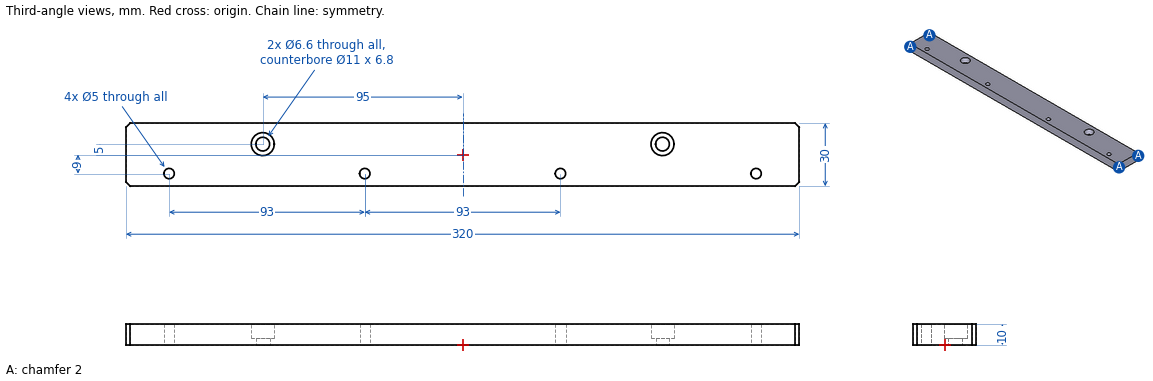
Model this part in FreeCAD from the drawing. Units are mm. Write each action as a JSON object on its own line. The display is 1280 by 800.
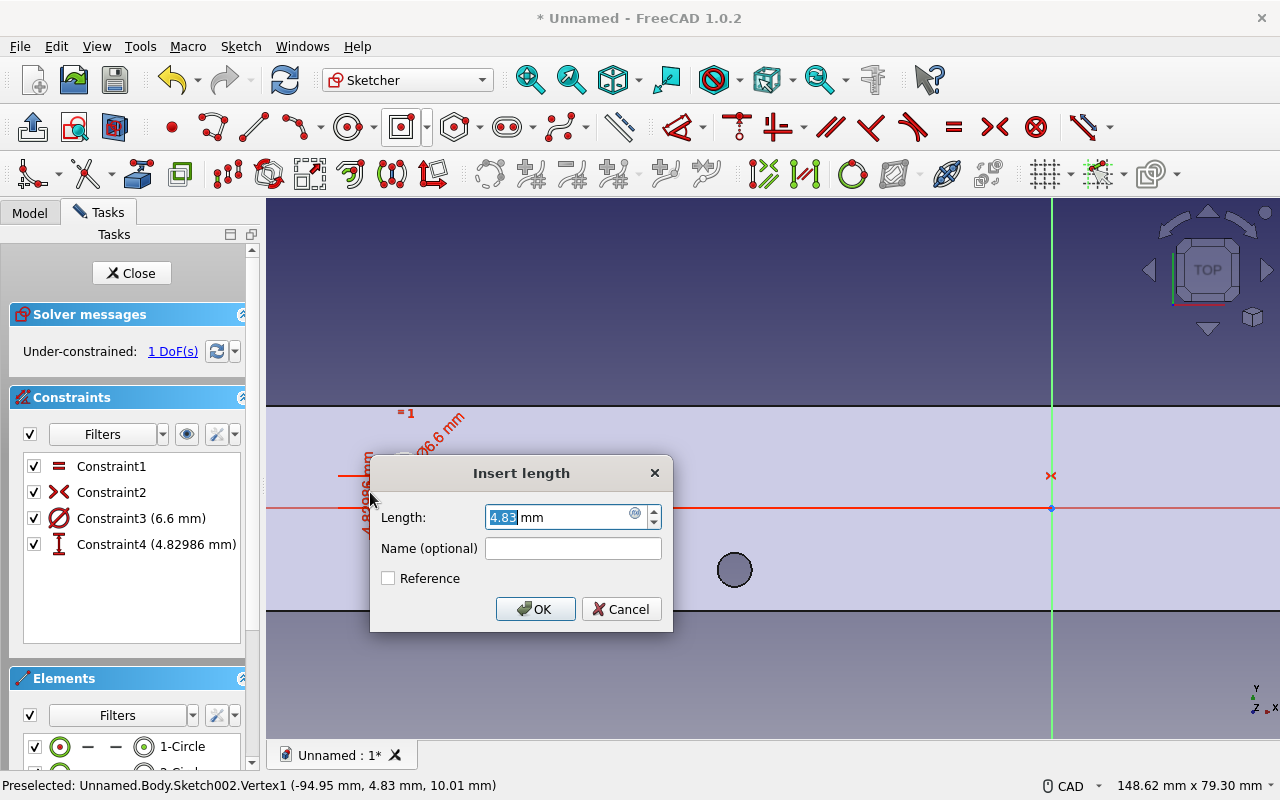
{"action": "type", "text": "5"}
{"action": "key", "text": "Return"}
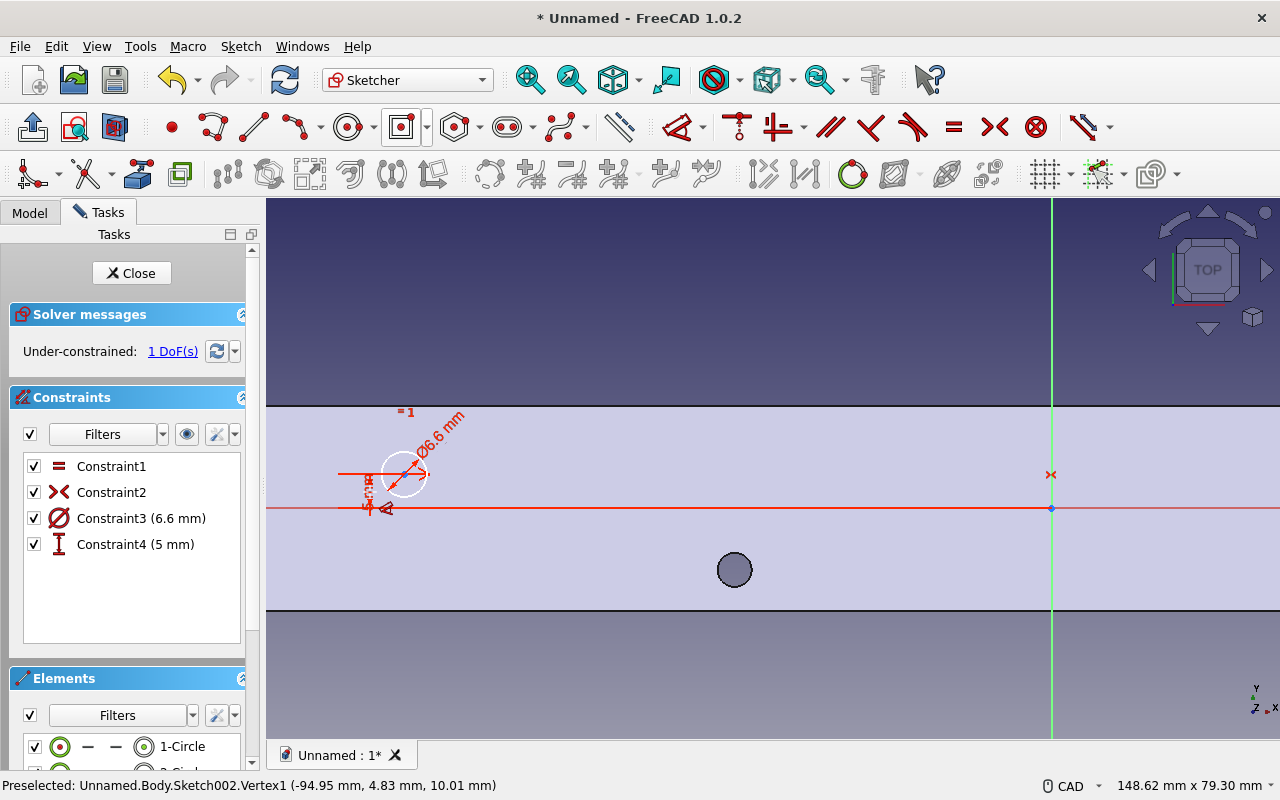
{"action": "left_click", "coordinate": [404, 474]}
{"action": "left_click", "coordinate": [728, 542]}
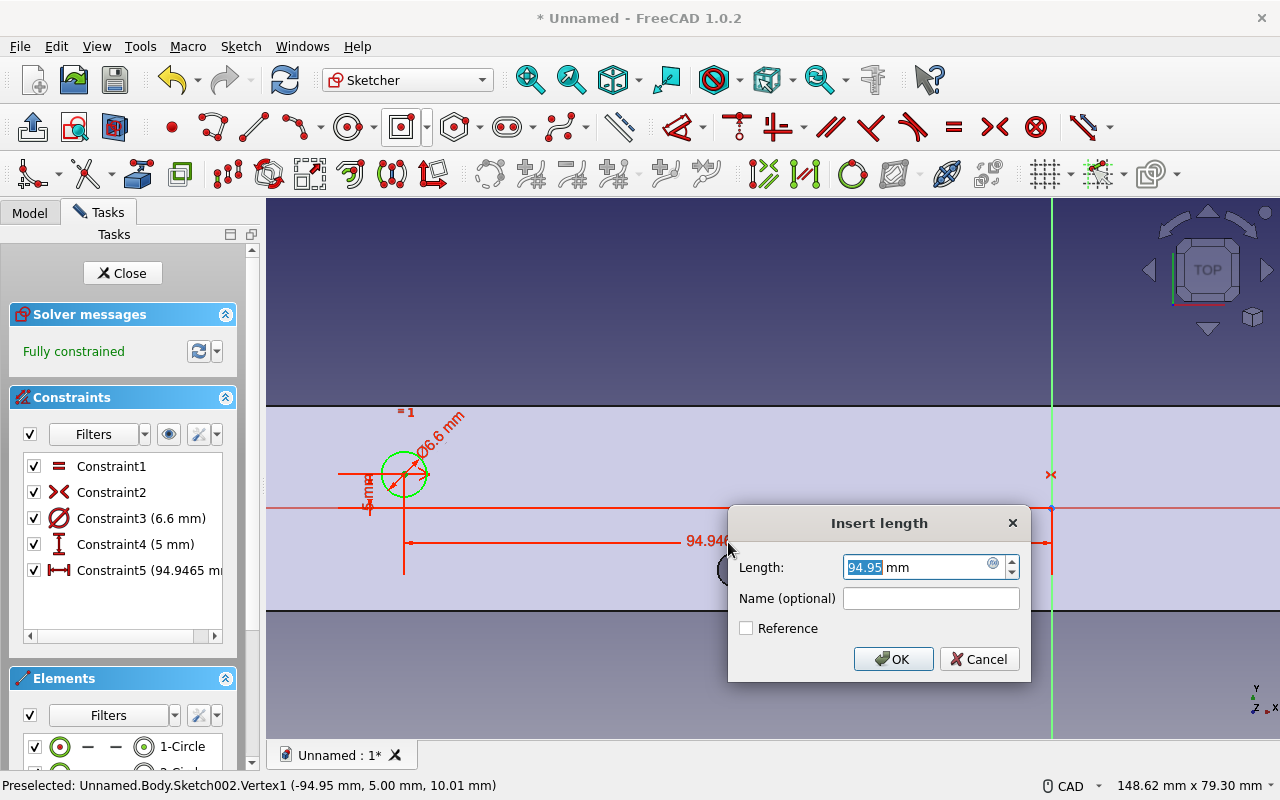
{"action": "type", "text": "95"}
{"action": "key", "text": "Return"}
{"action": "key", "text": "Escape"}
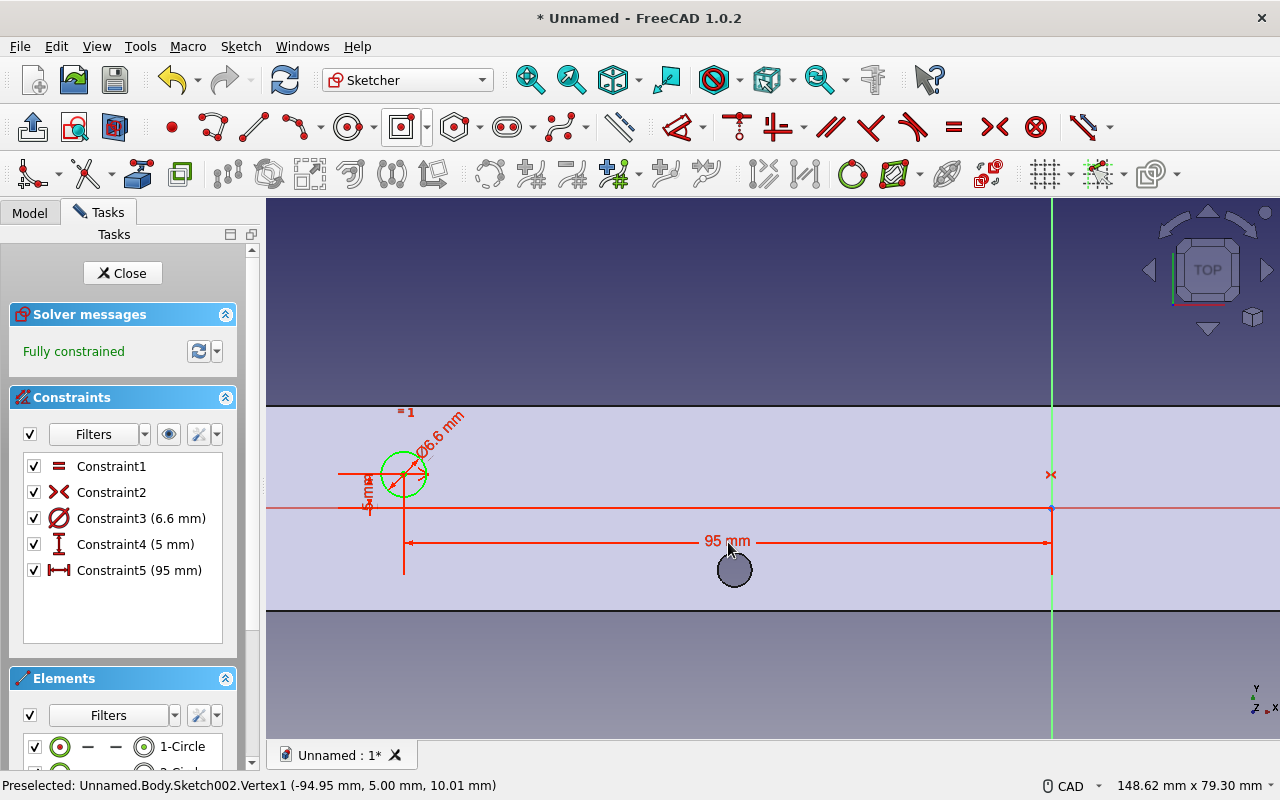
{"action": "left_click", "coordinate": [123, 273]}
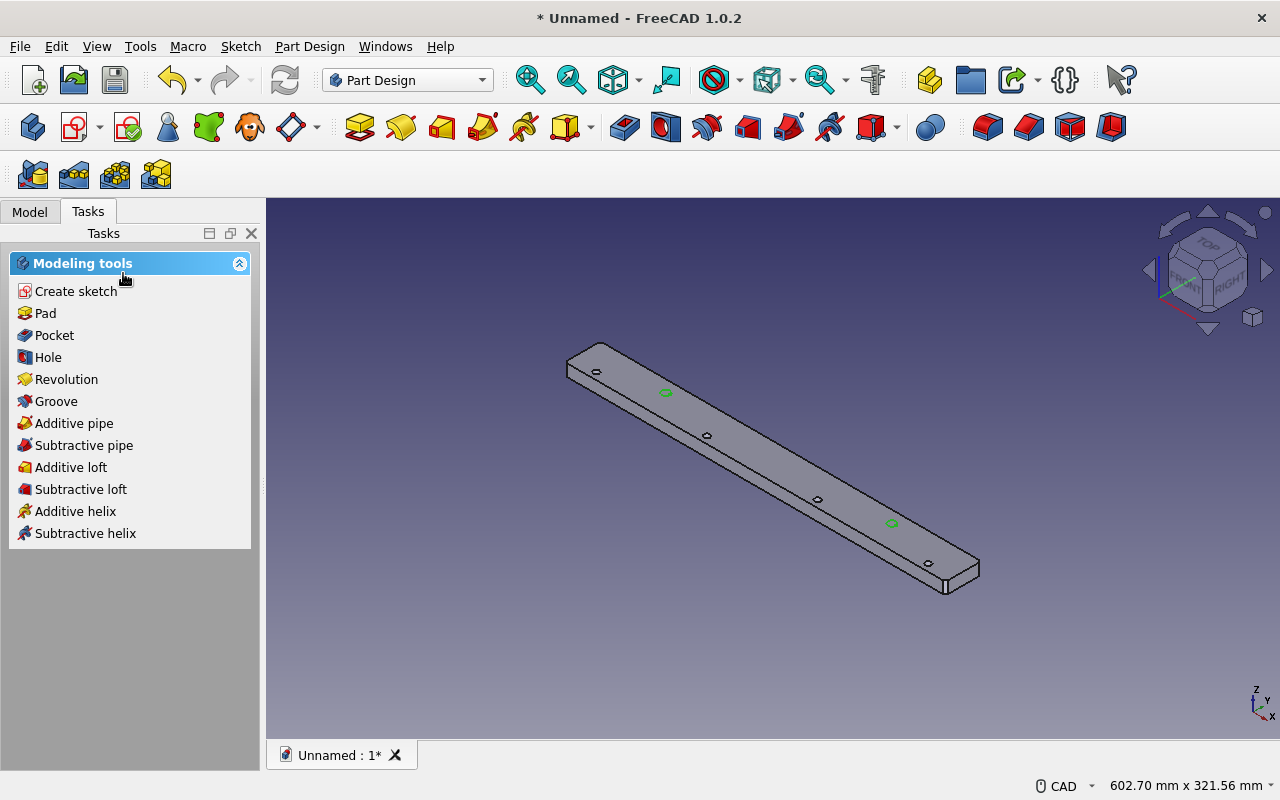
{"action": "left_click", "coordinate": [666, 128]}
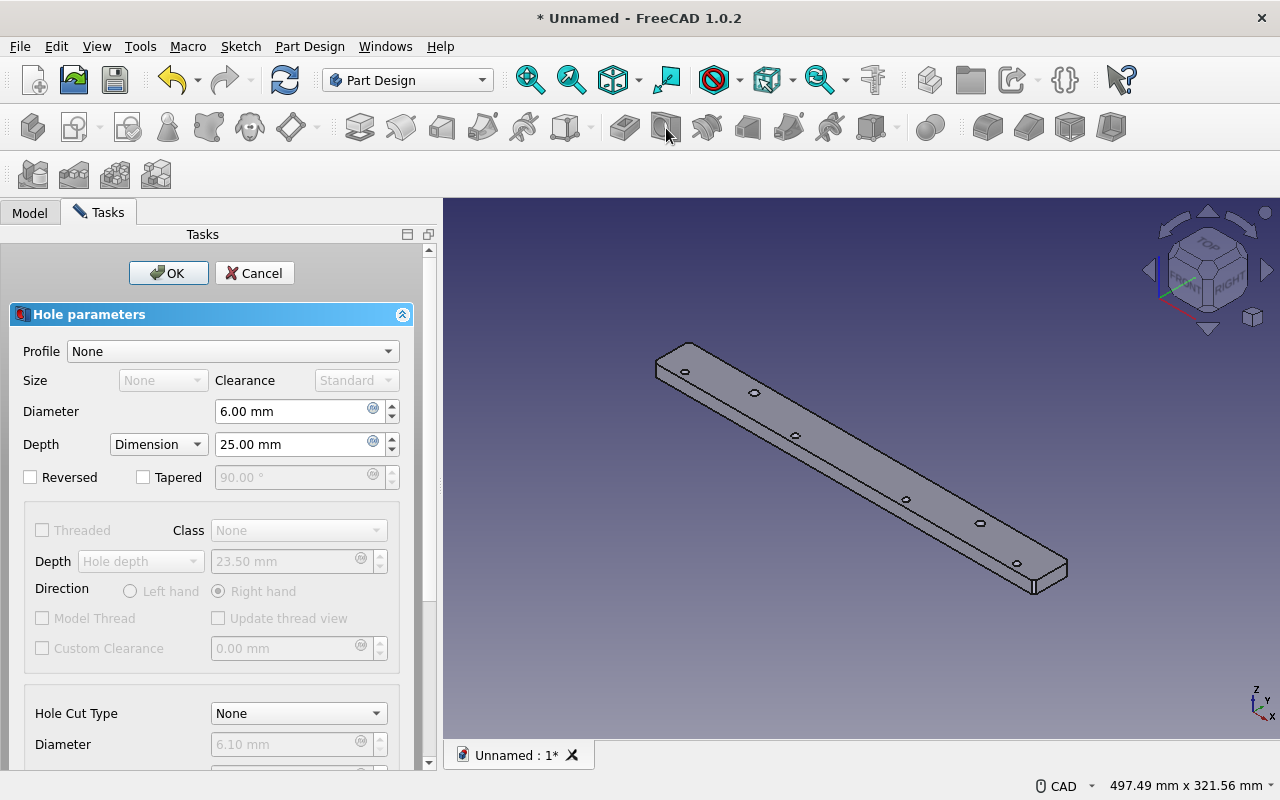
{"action": "triple_click", "coordinate": [300, 412]}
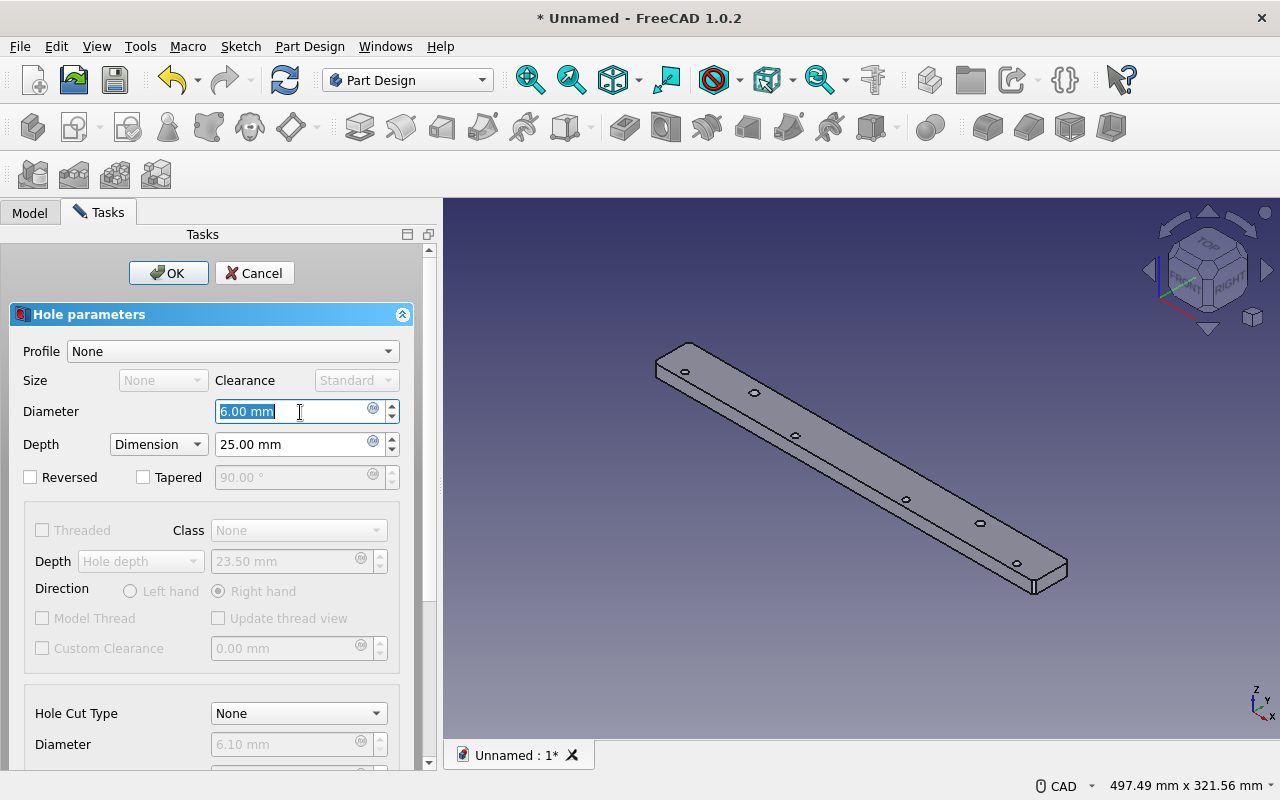
{"action": "type", "text": "6.6"}
{"action": "key", "text": "Tab"}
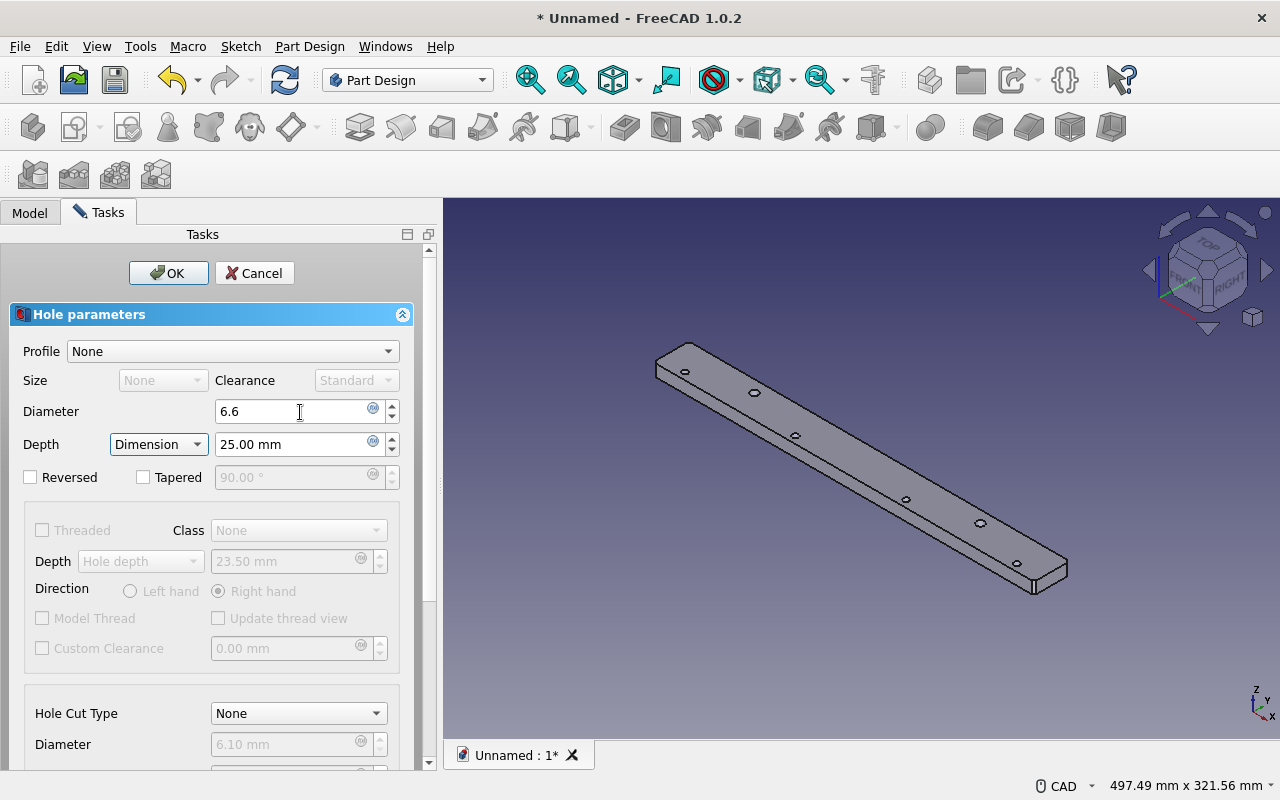
{"action": "left_click", "coordinate": [160, 444]}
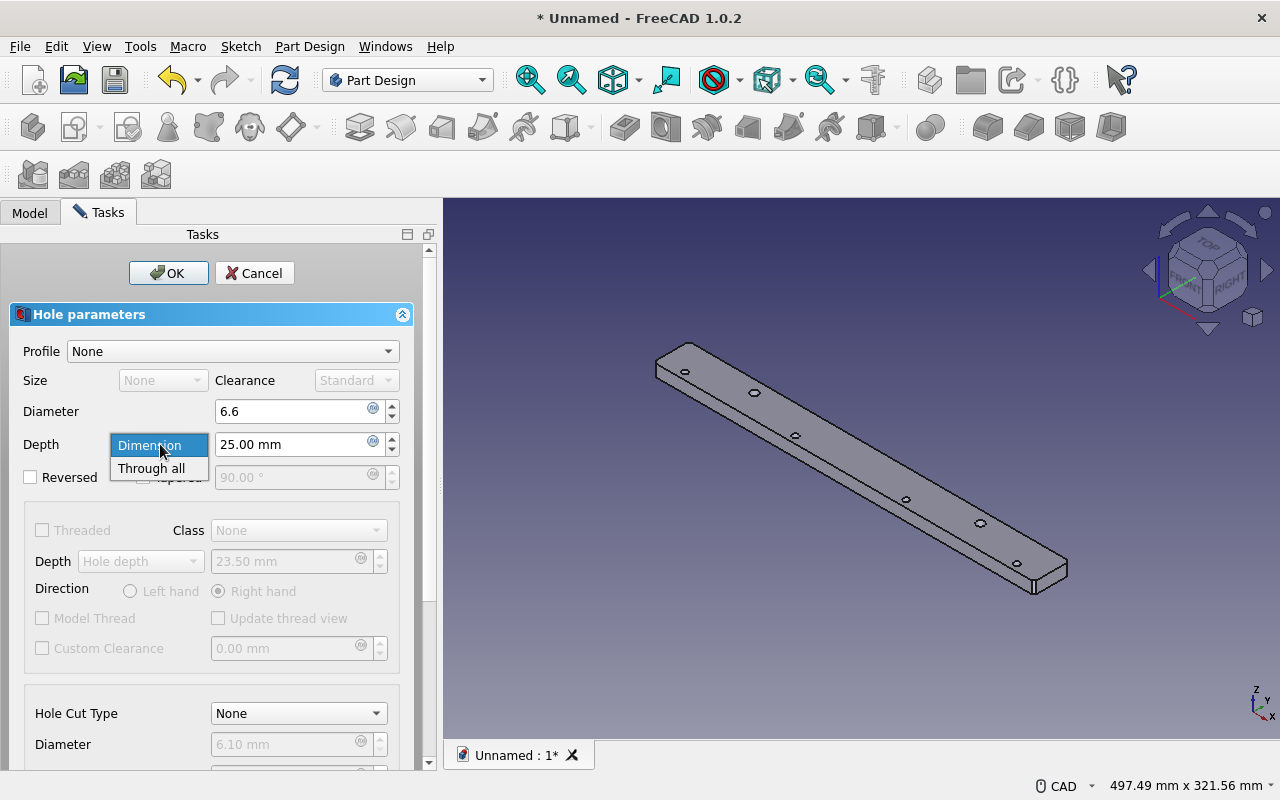
{"action": "left_click", "coordinate": [158, 468]}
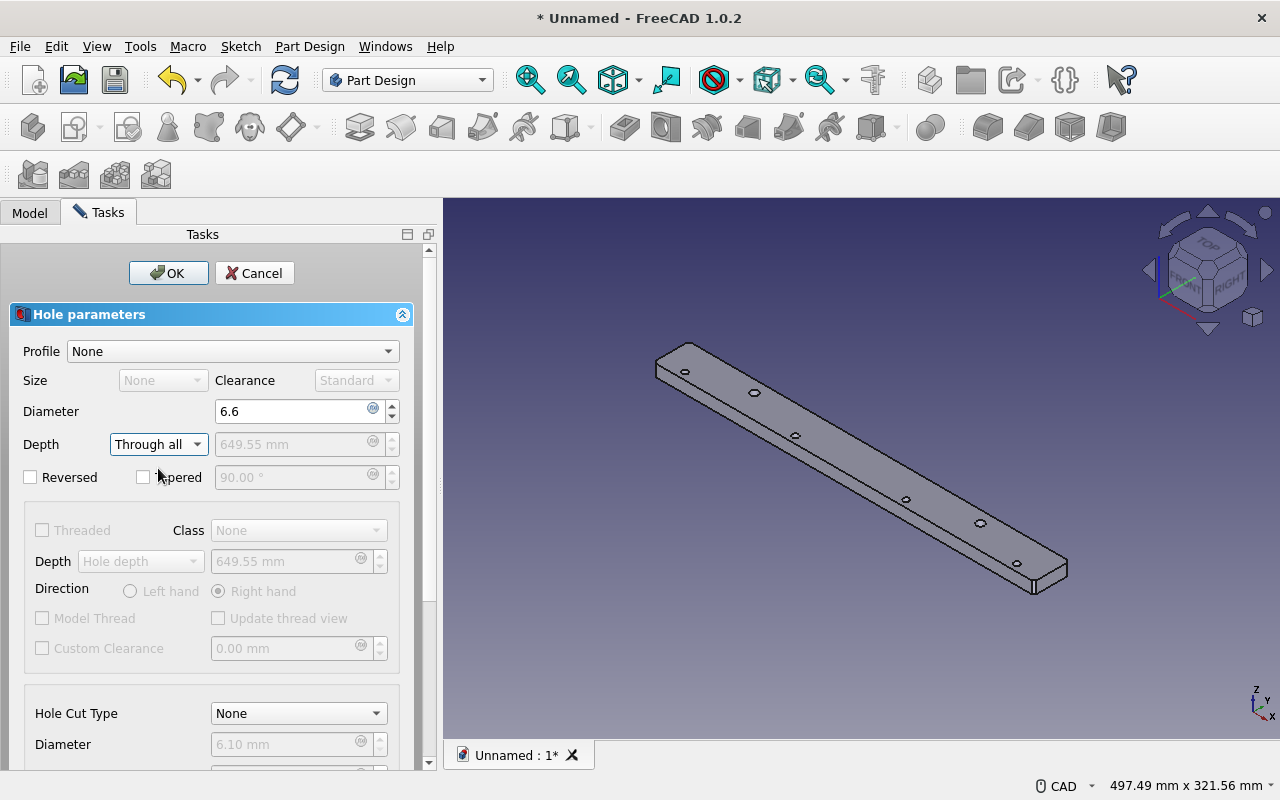
{"action": "left_click", "coordinate": [300, 714]}